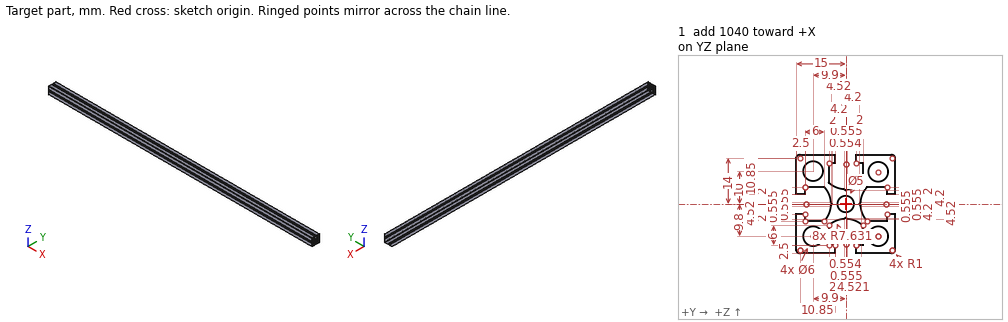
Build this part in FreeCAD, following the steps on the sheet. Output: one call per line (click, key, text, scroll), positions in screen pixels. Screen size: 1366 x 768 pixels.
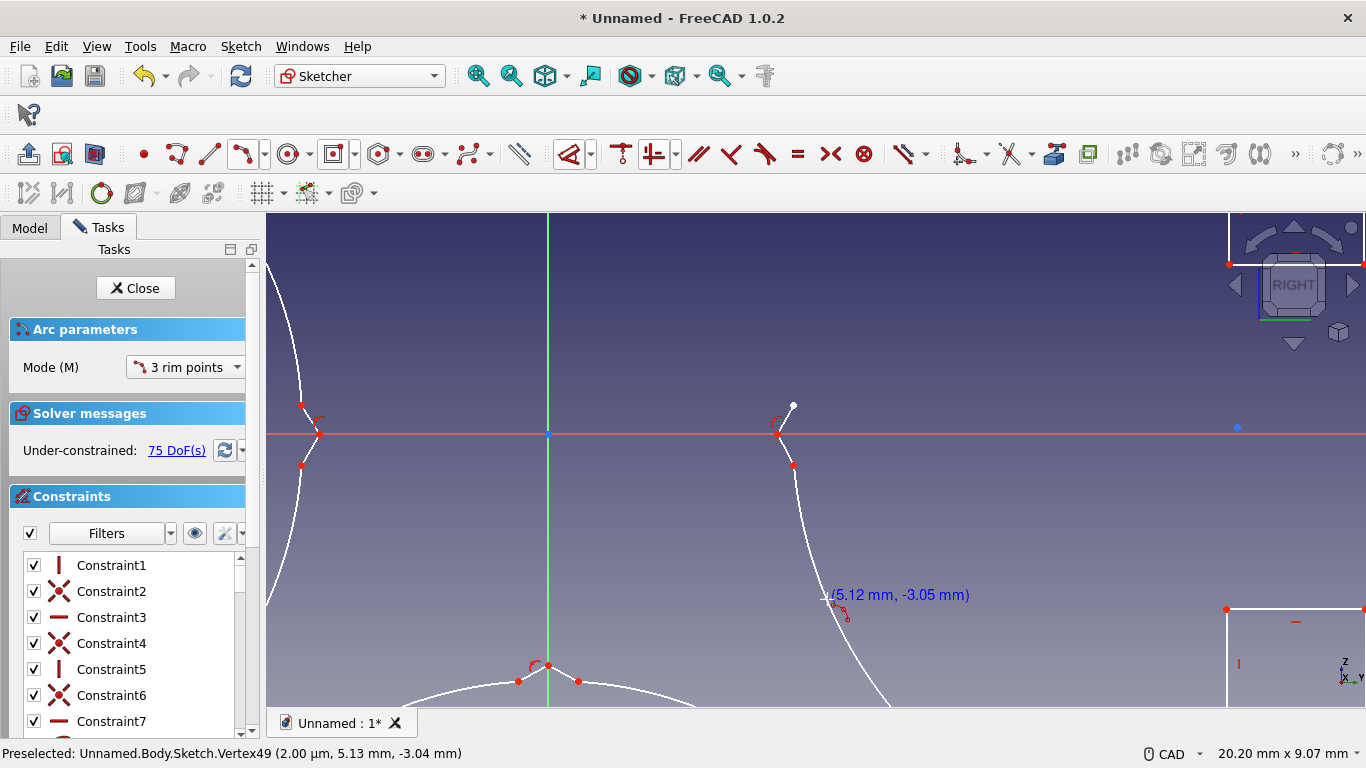
click(794, 405)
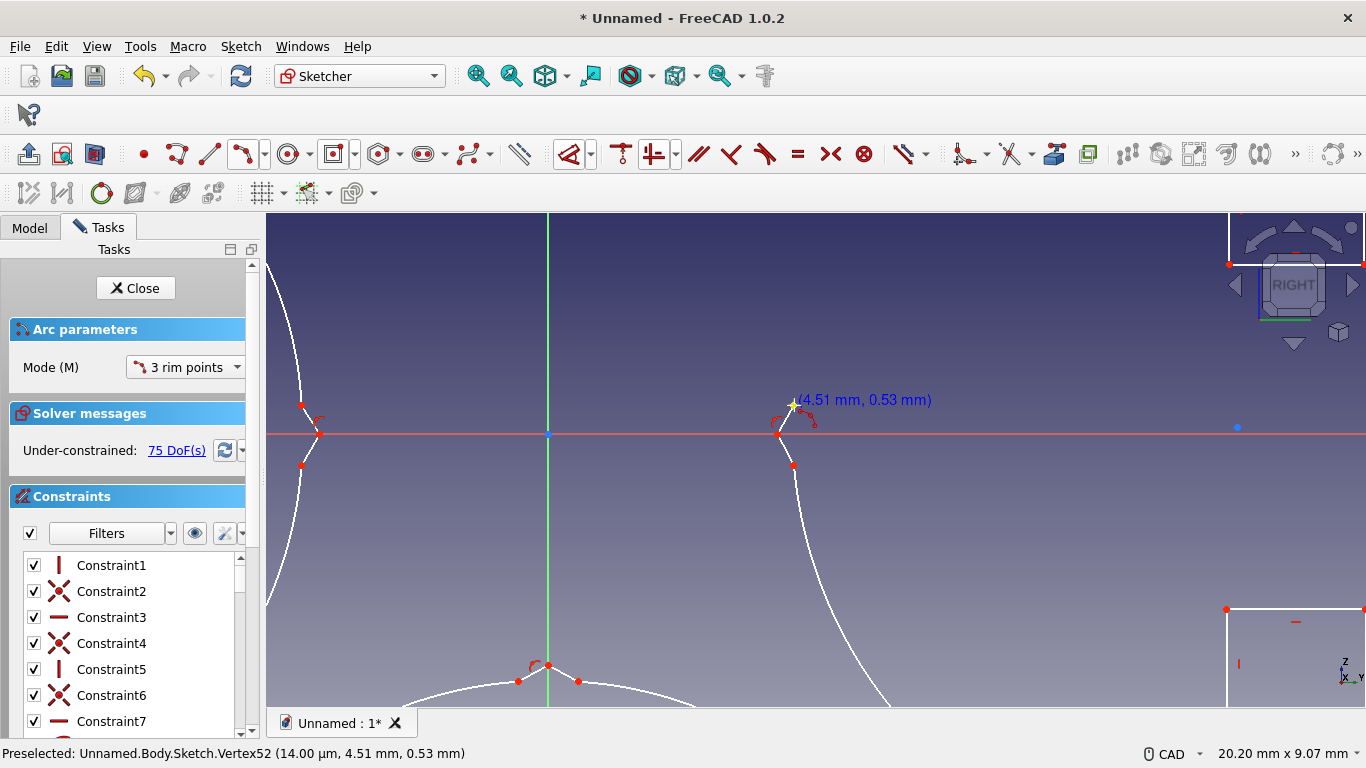
scroll(798, 467, down, 8)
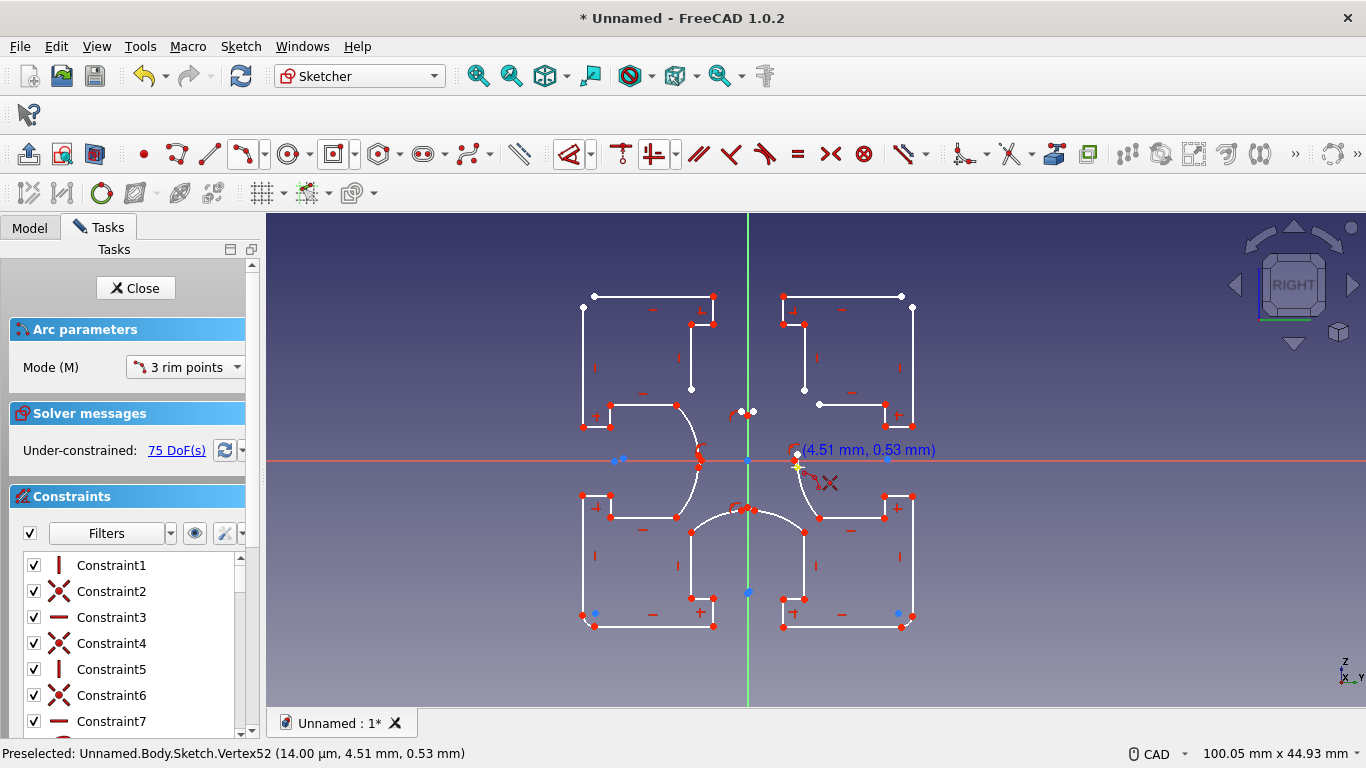
click(819, 405)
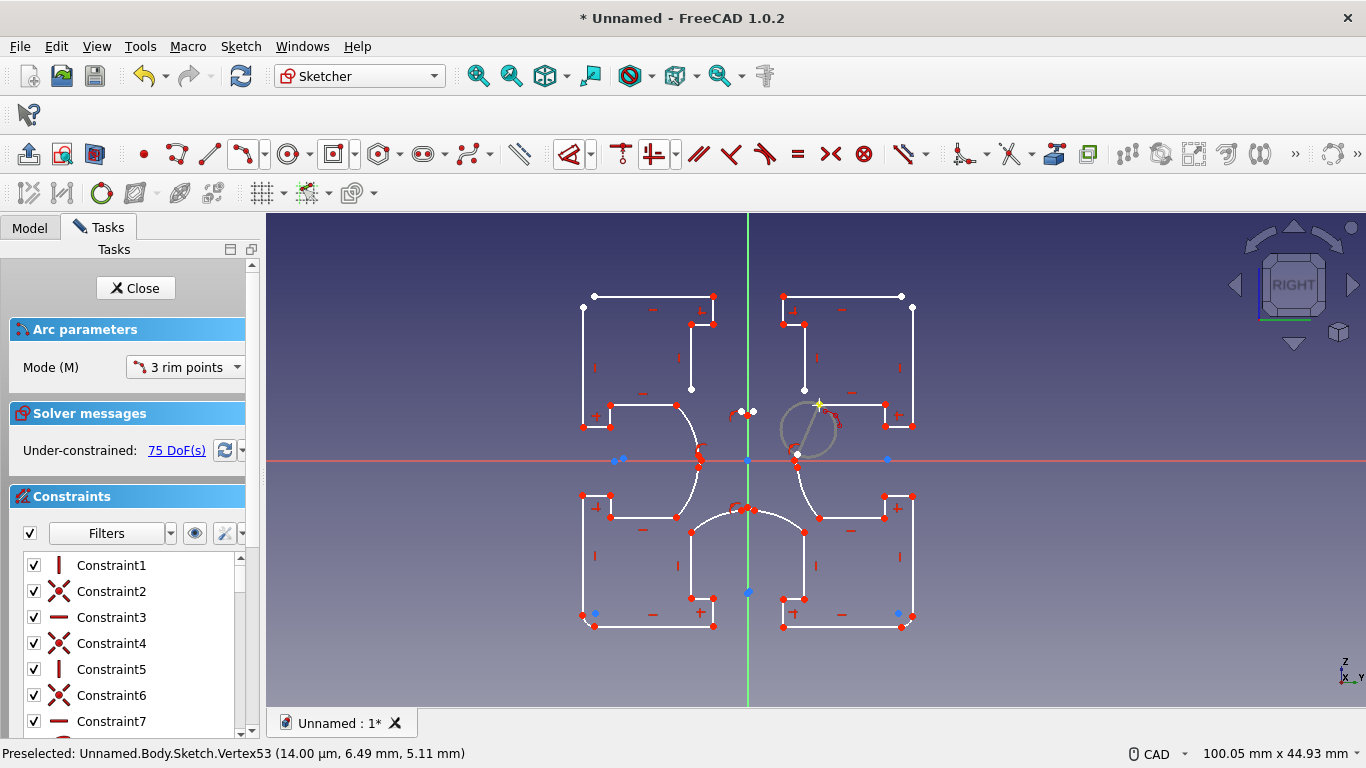
scroll(804, 428, up, 7)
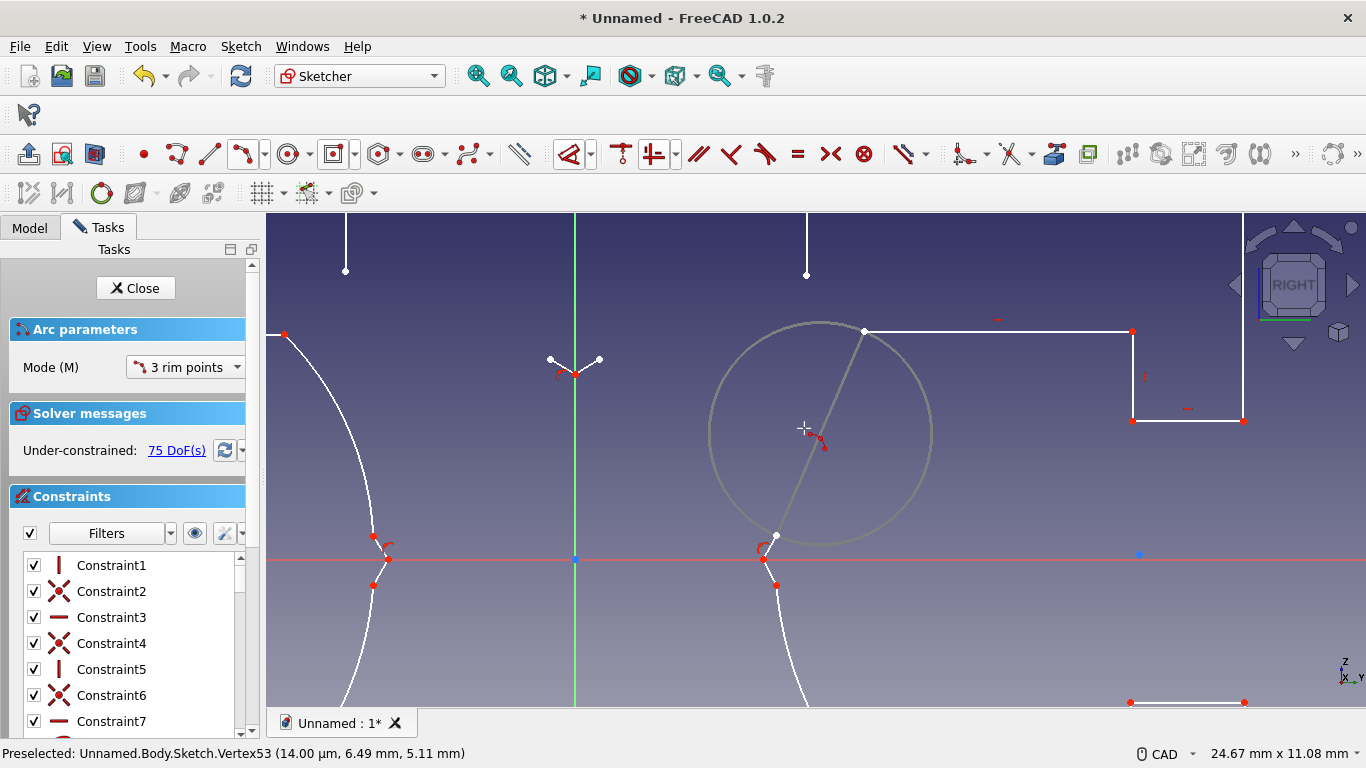
click(804, 425)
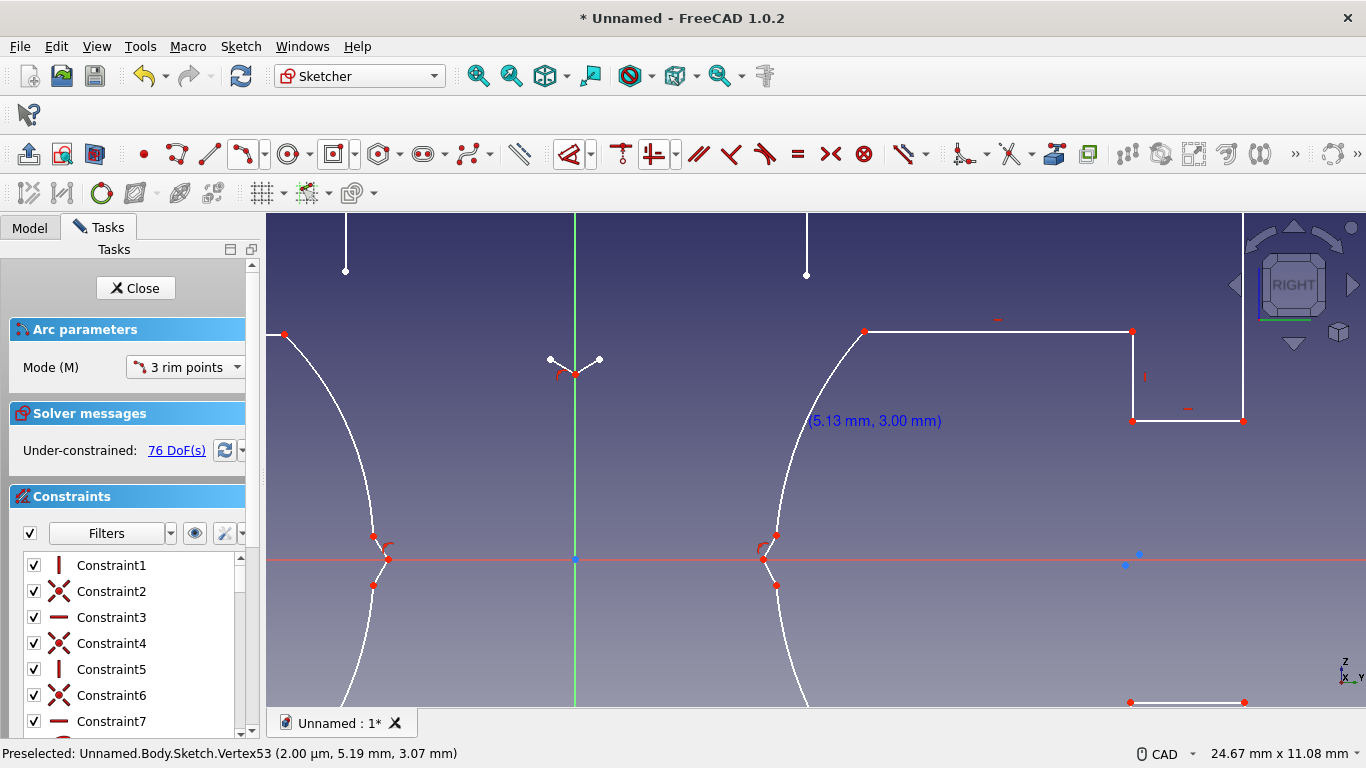
scroll(804, 427, down, 7)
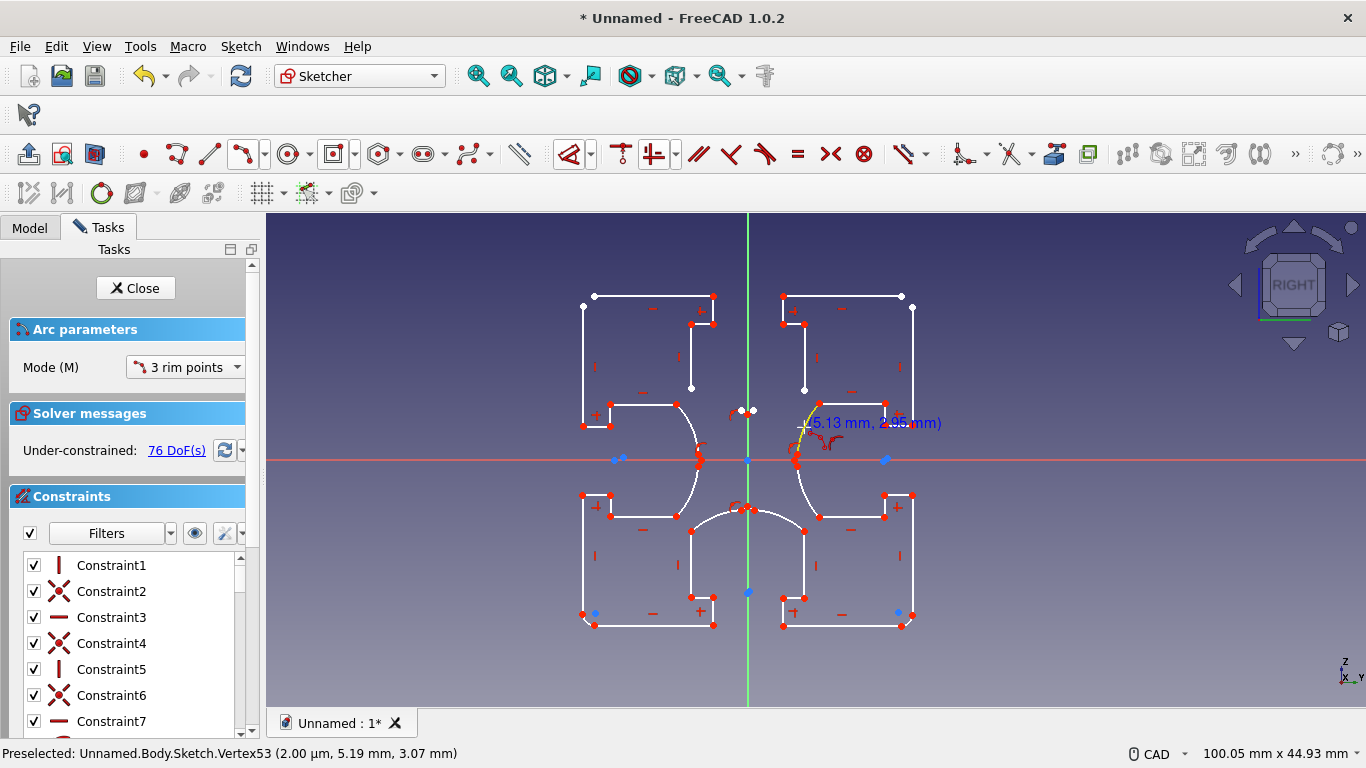
click(913, 307)
click(902, 296)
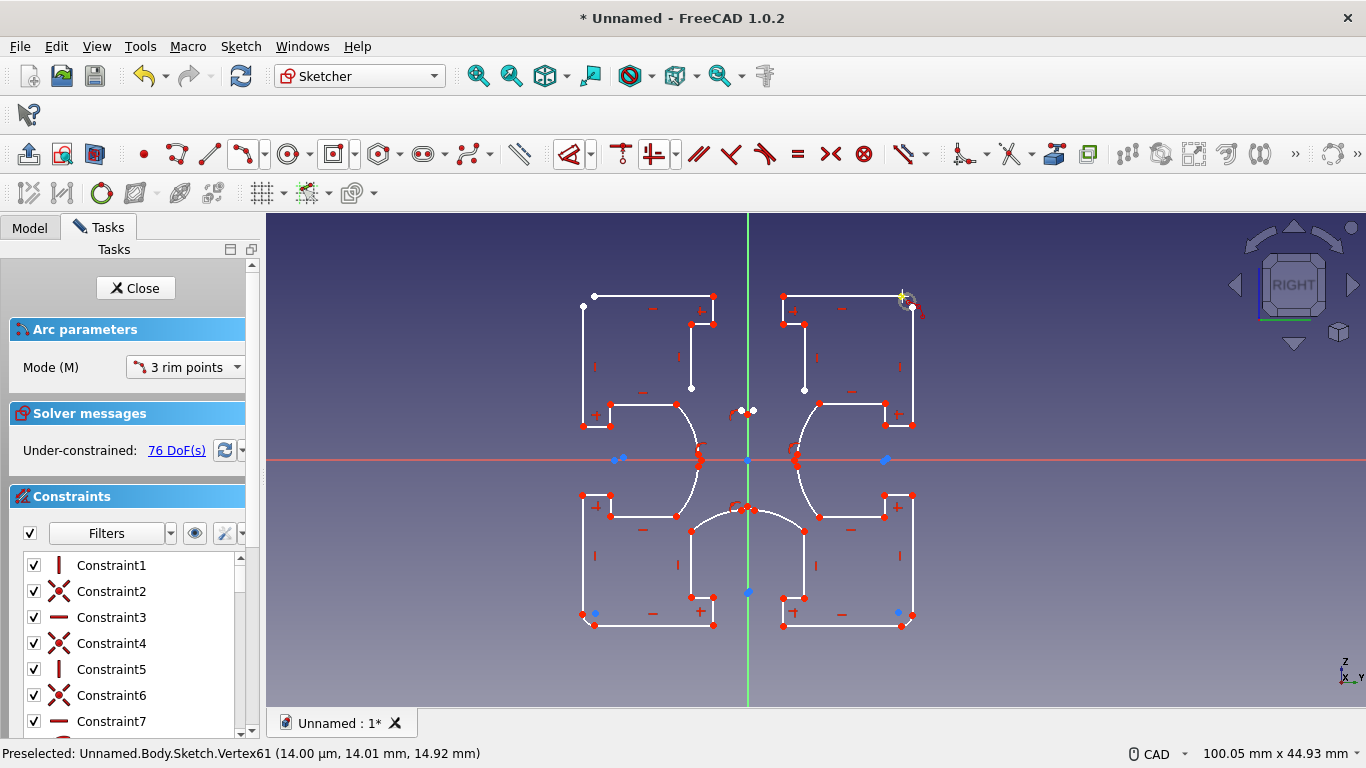
scroll(910, 298, up, 8)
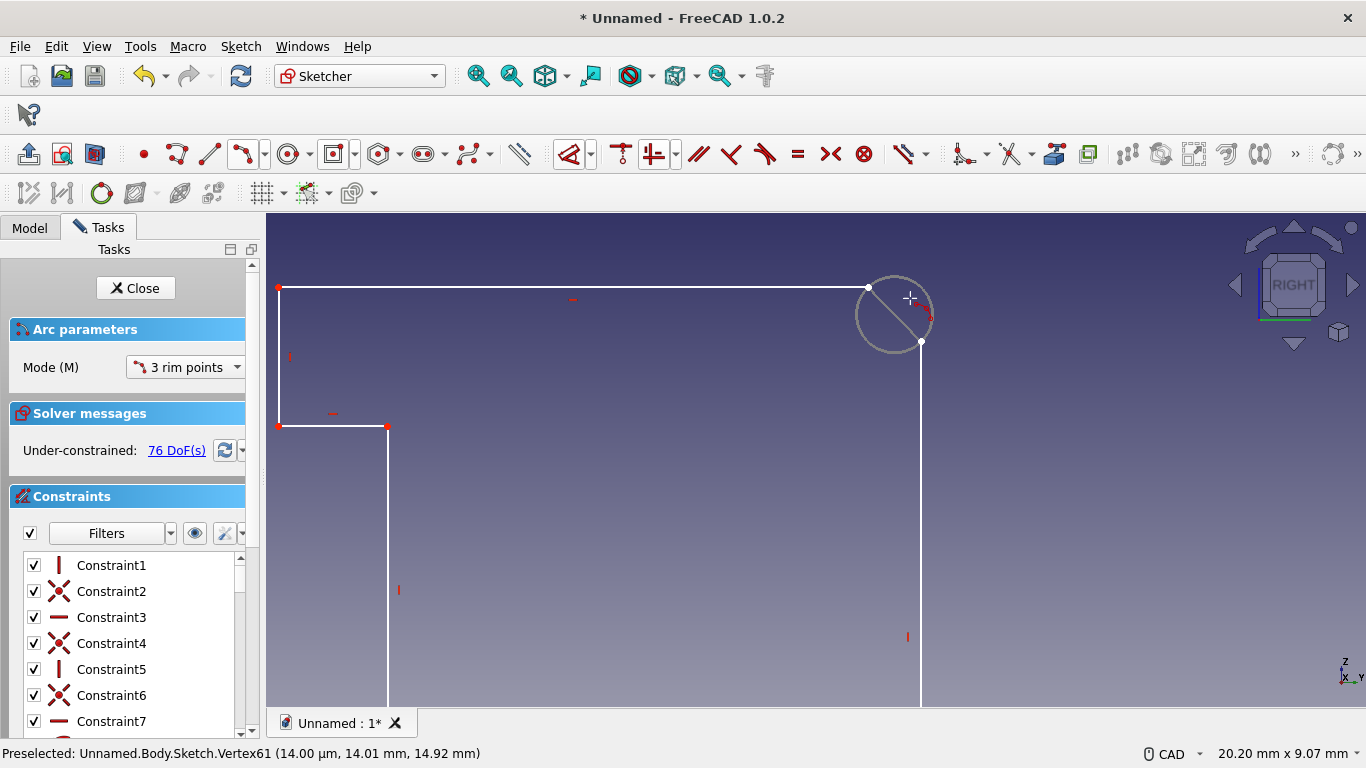
click(906, 299)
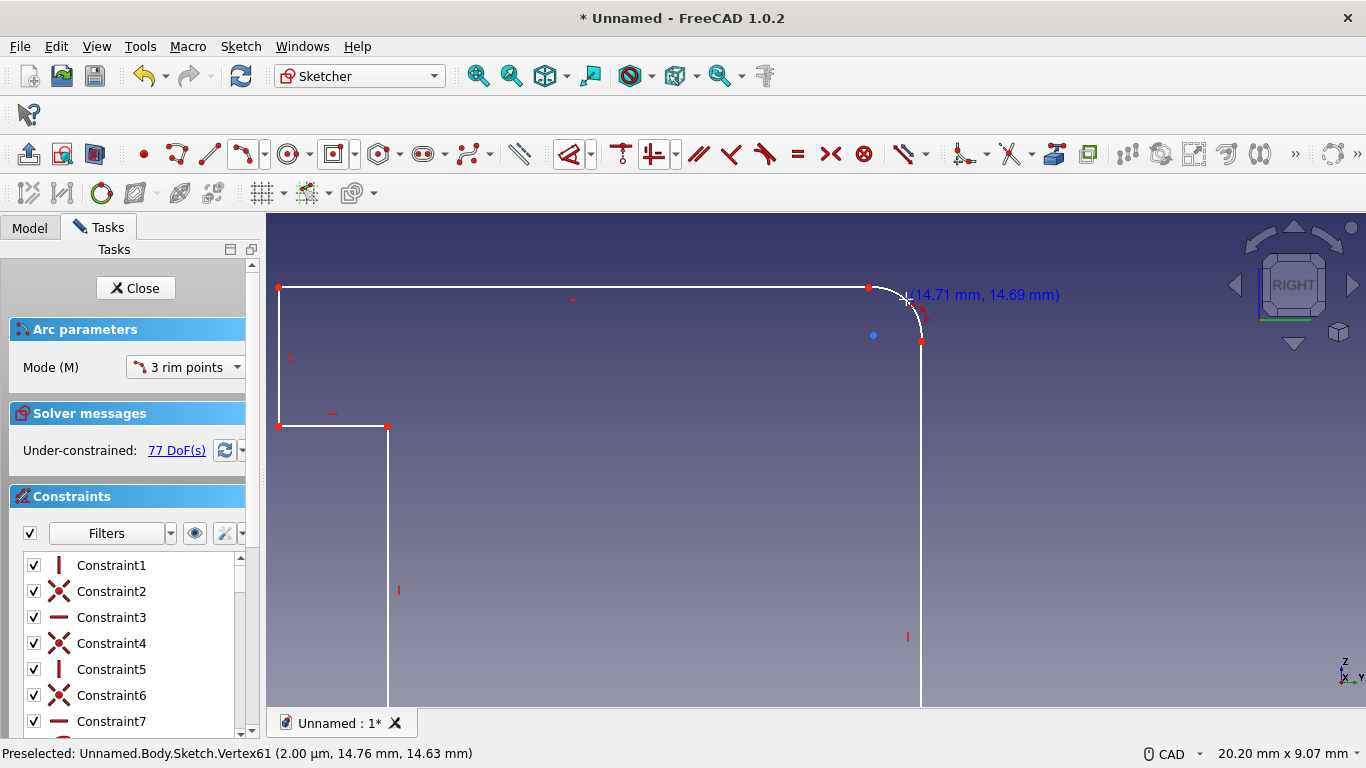
scroll(910, 298, down, 8)